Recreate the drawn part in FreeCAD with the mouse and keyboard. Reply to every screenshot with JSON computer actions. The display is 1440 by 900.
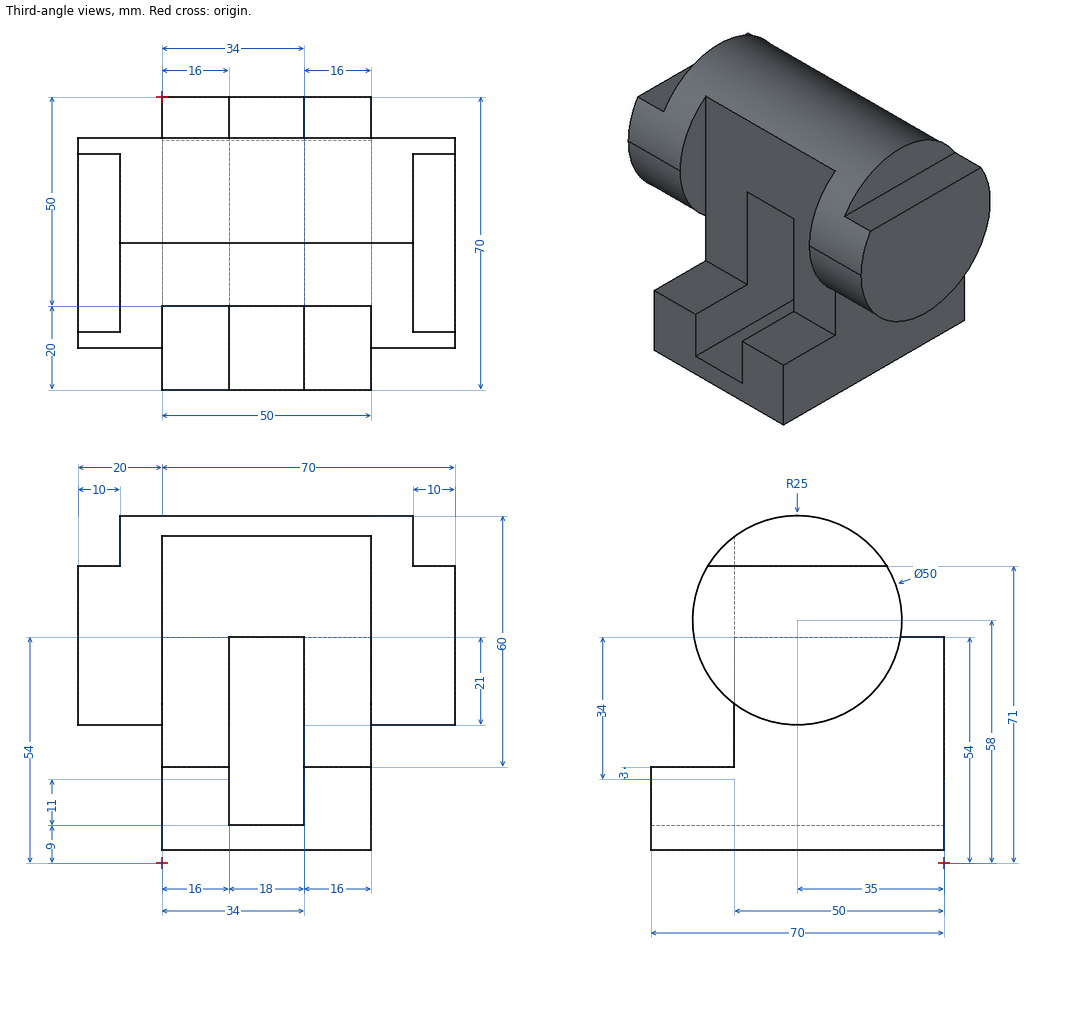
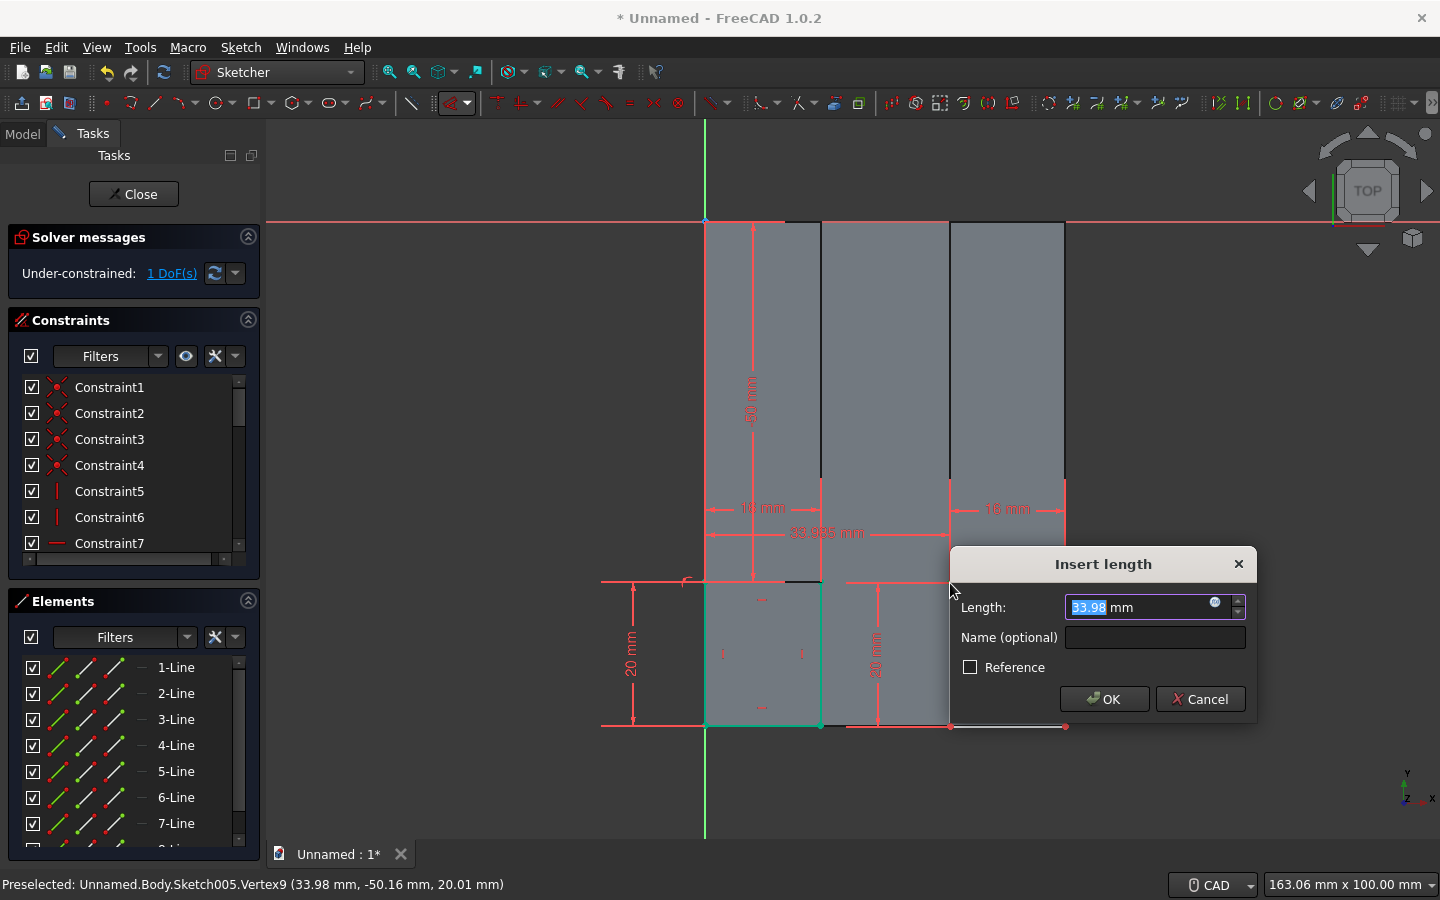
{"action": "type", "text": "34"}
{"action": "key", "text": "Return"}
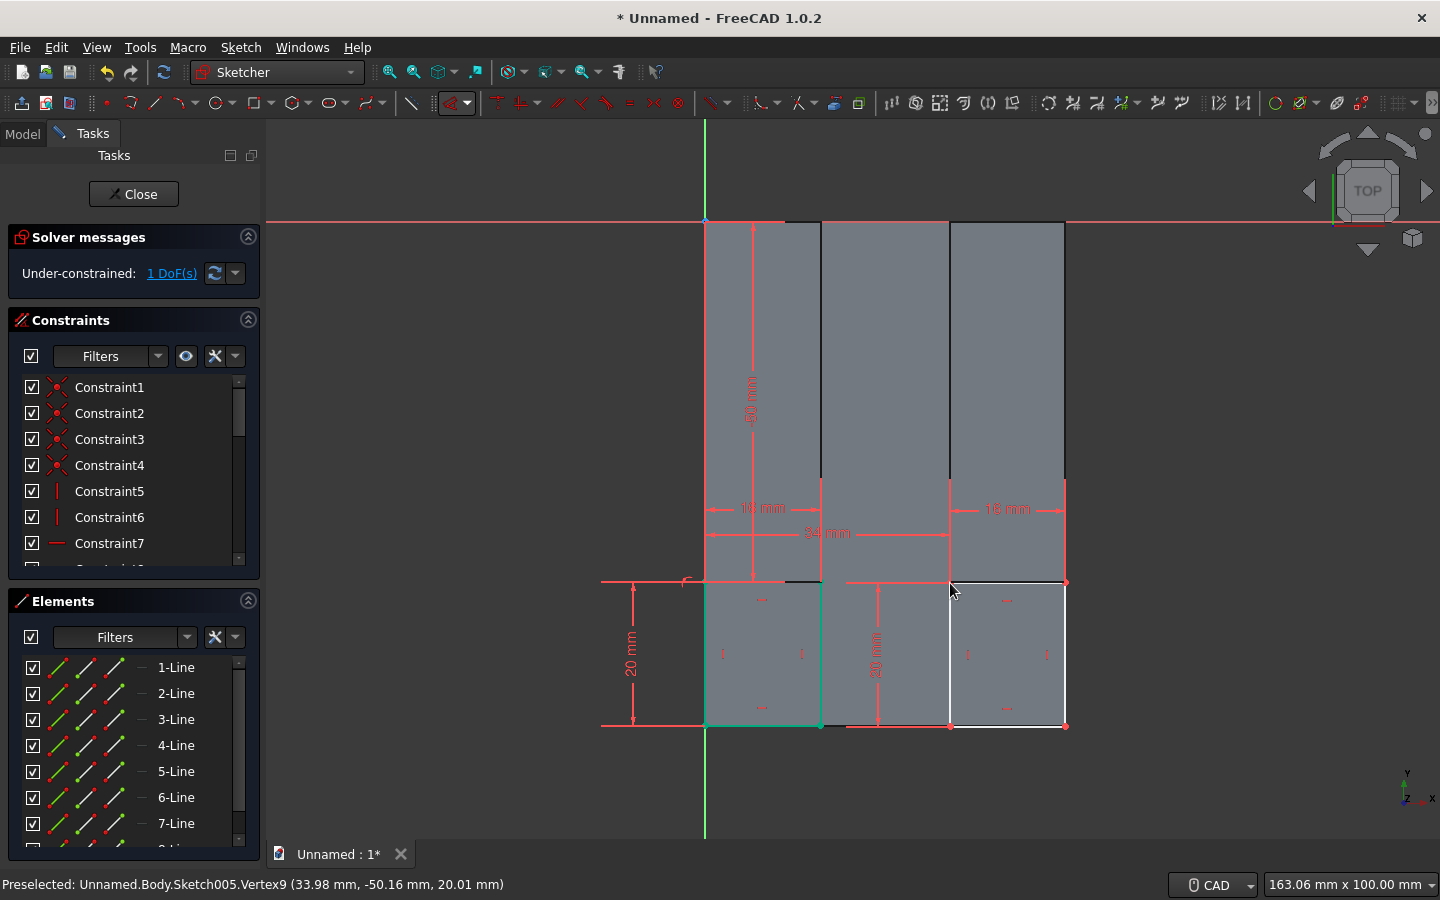
{"action": "left_click", "coordinate": [950, 583]}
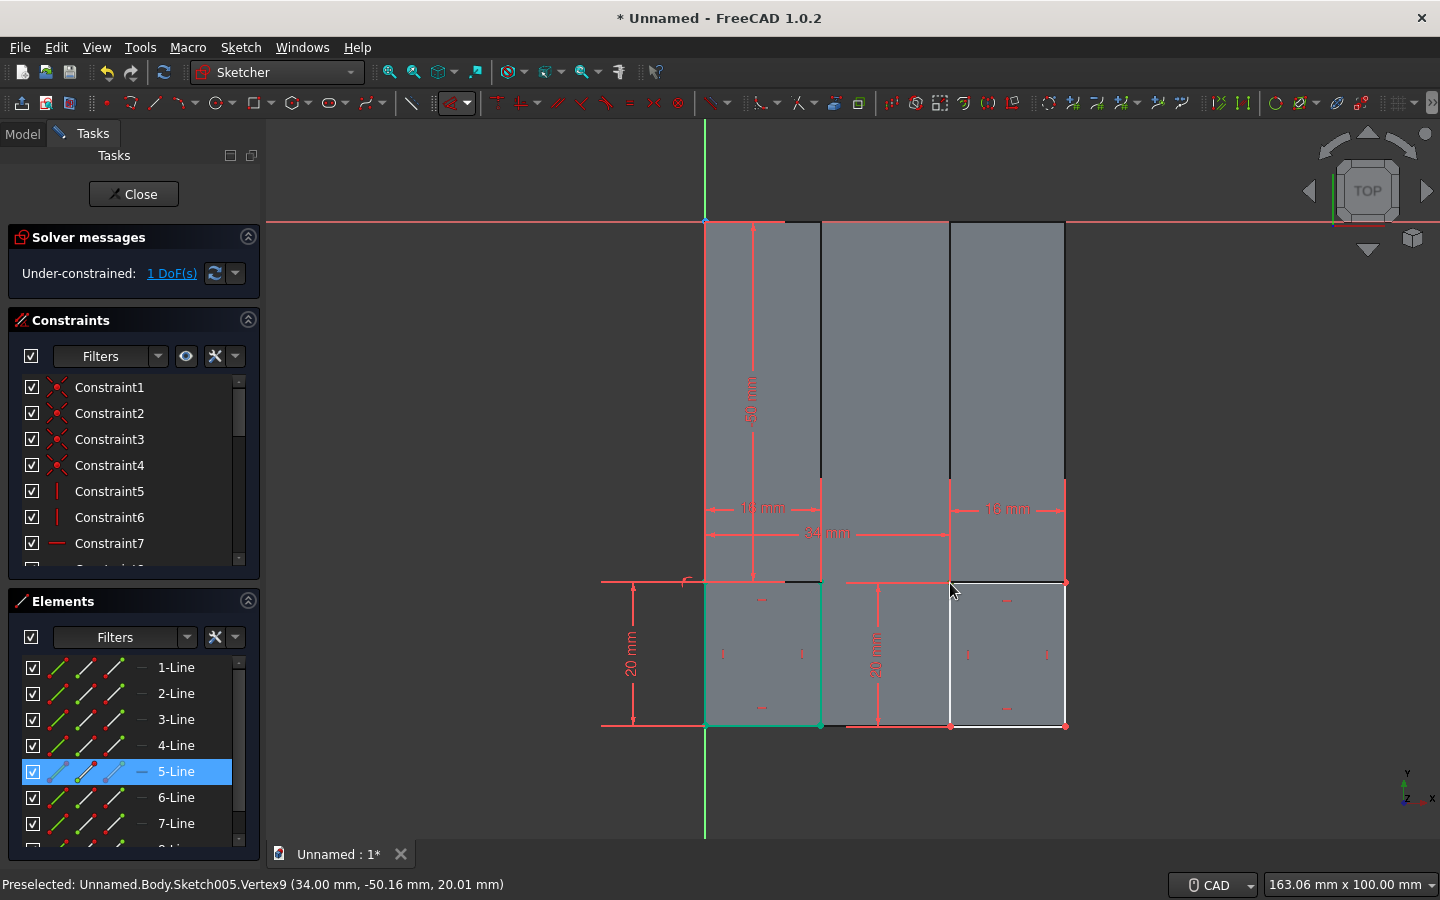
{"action": "key", "text": "i"}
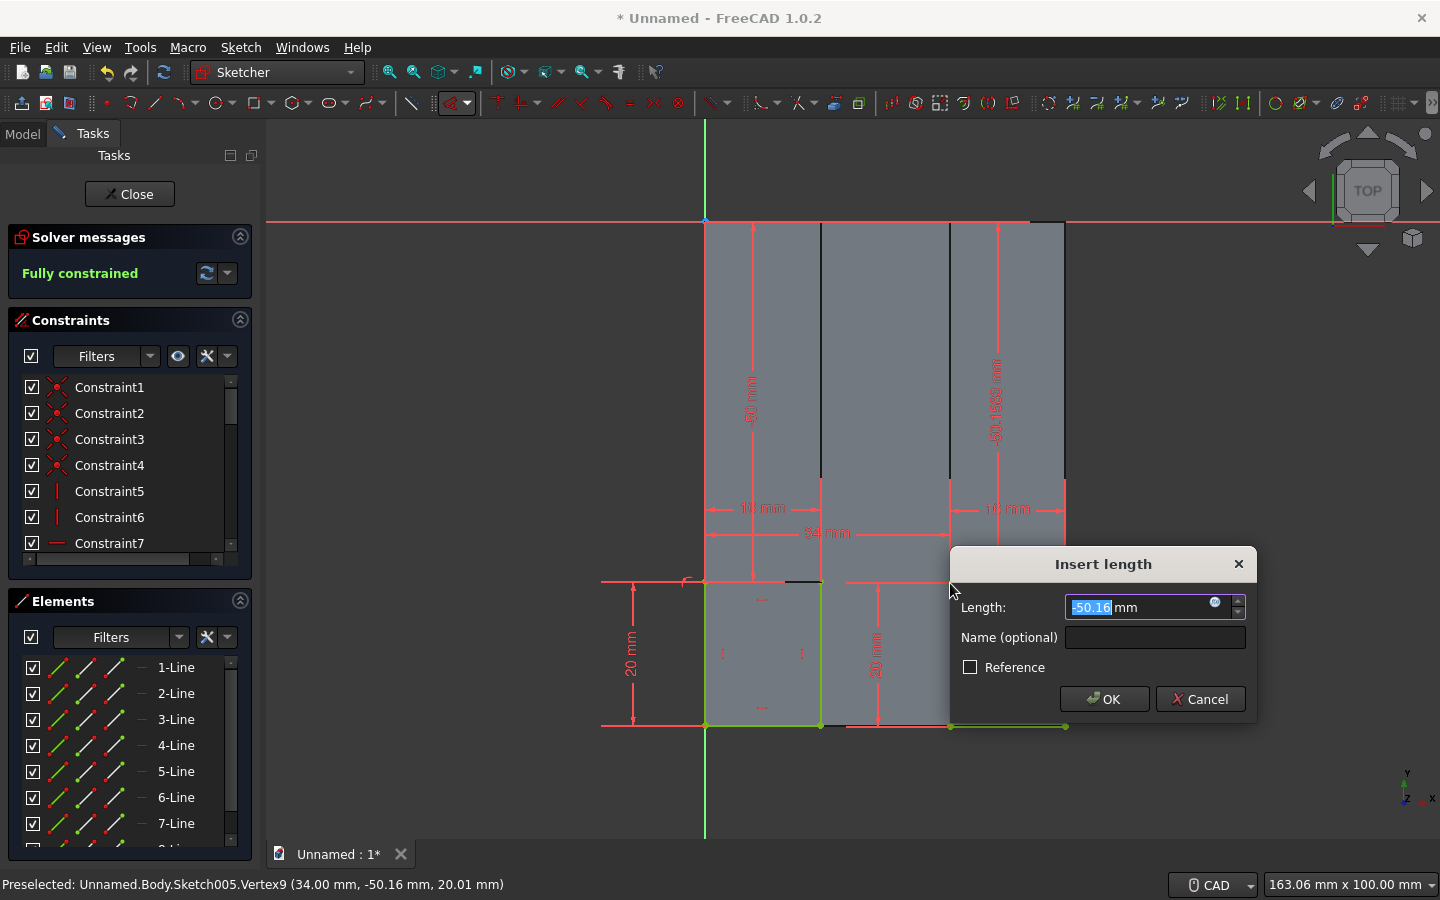
{"action": "type", "text": "-50"}
{"action": "key", "text": "Return"}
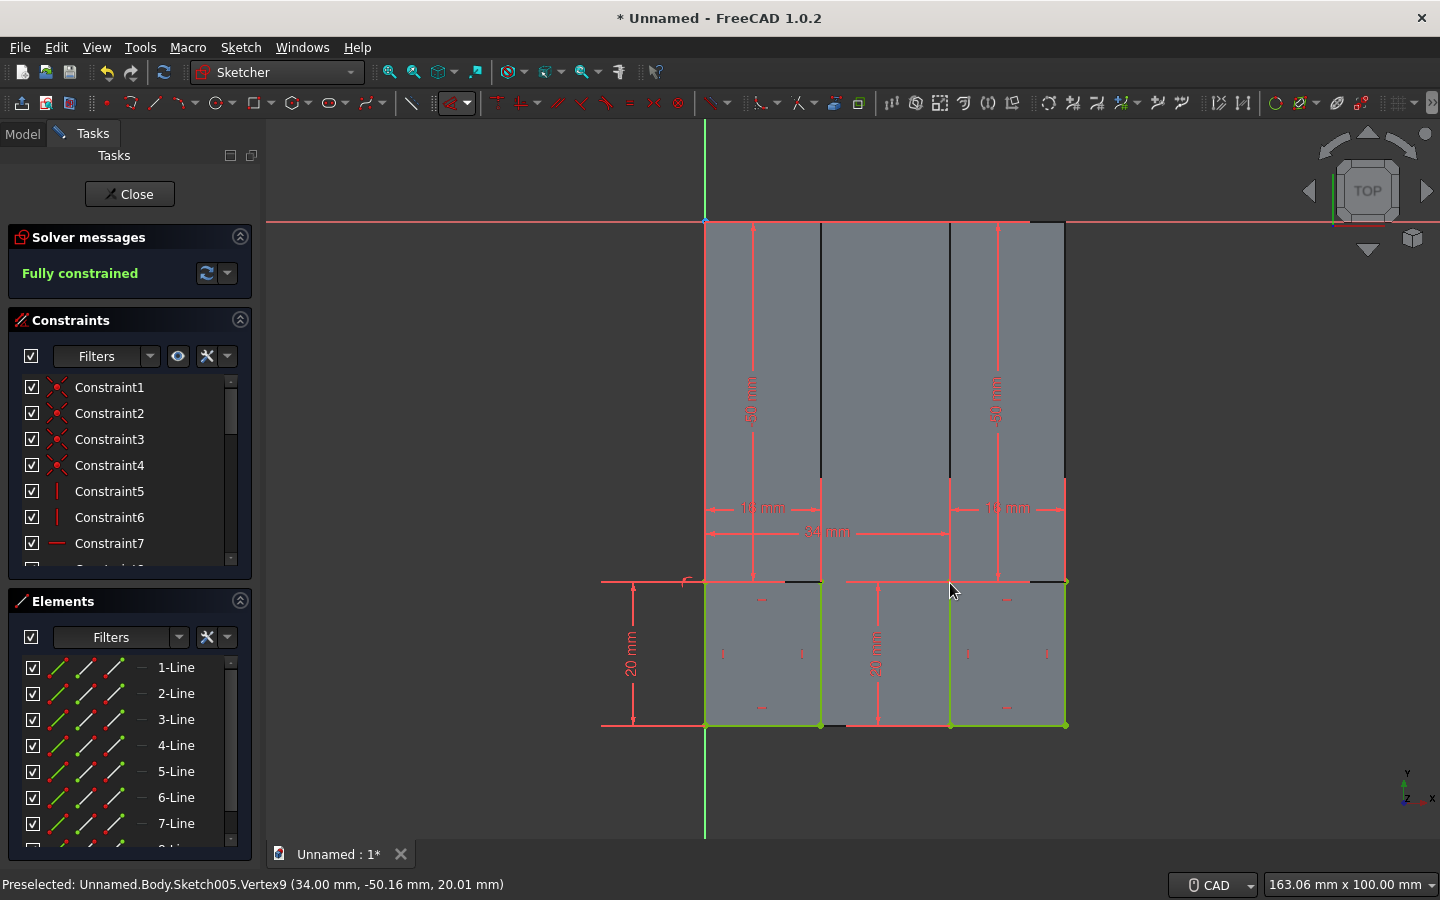
{"action": "left_click", "coordinate": [130, 194]}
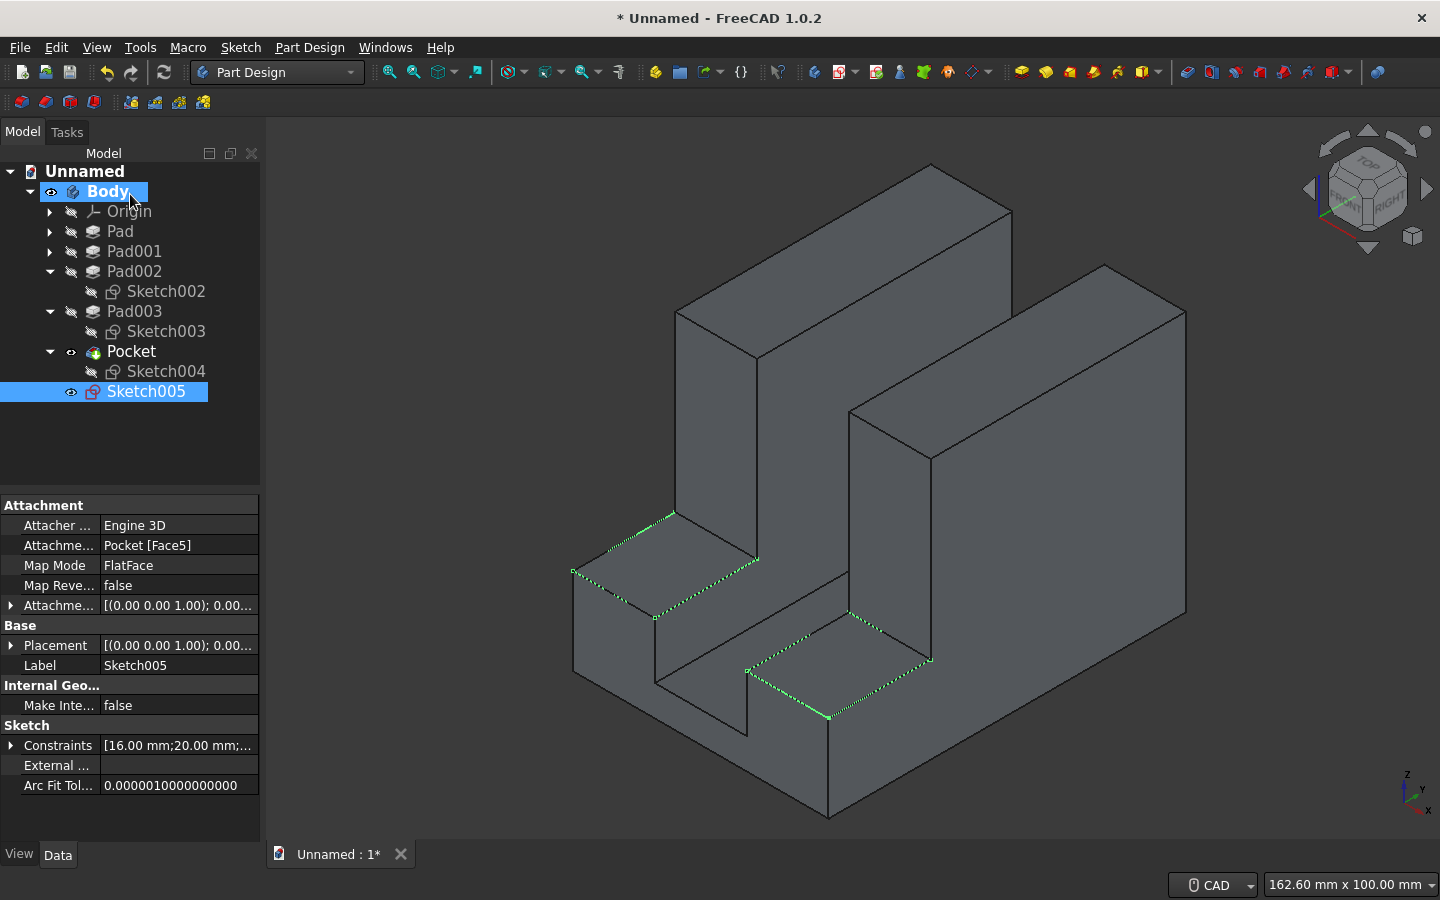
{"action": "left_click", "coordinate": [1022, 72]}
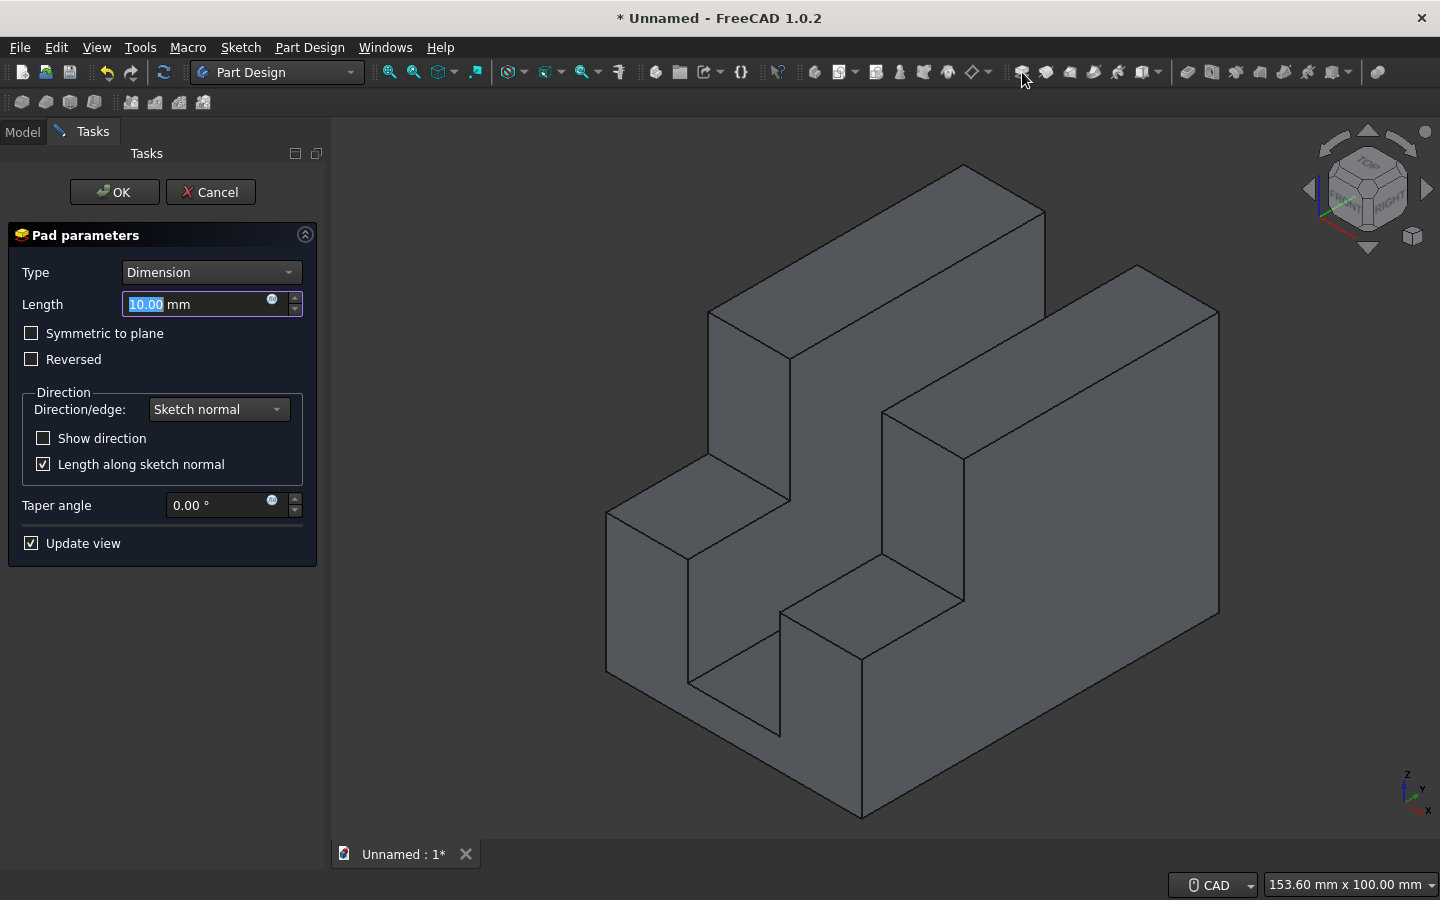
{"action": "type", "text": "3"}
{"action": "key", "text": "Tab"}